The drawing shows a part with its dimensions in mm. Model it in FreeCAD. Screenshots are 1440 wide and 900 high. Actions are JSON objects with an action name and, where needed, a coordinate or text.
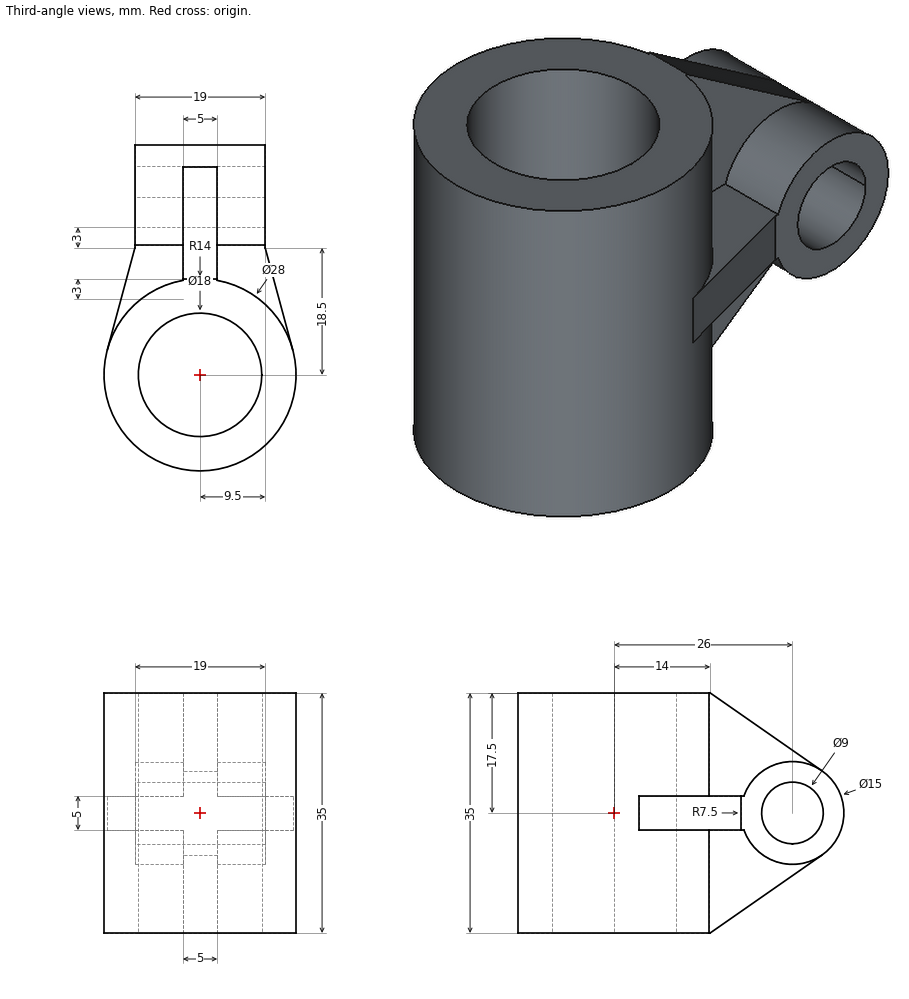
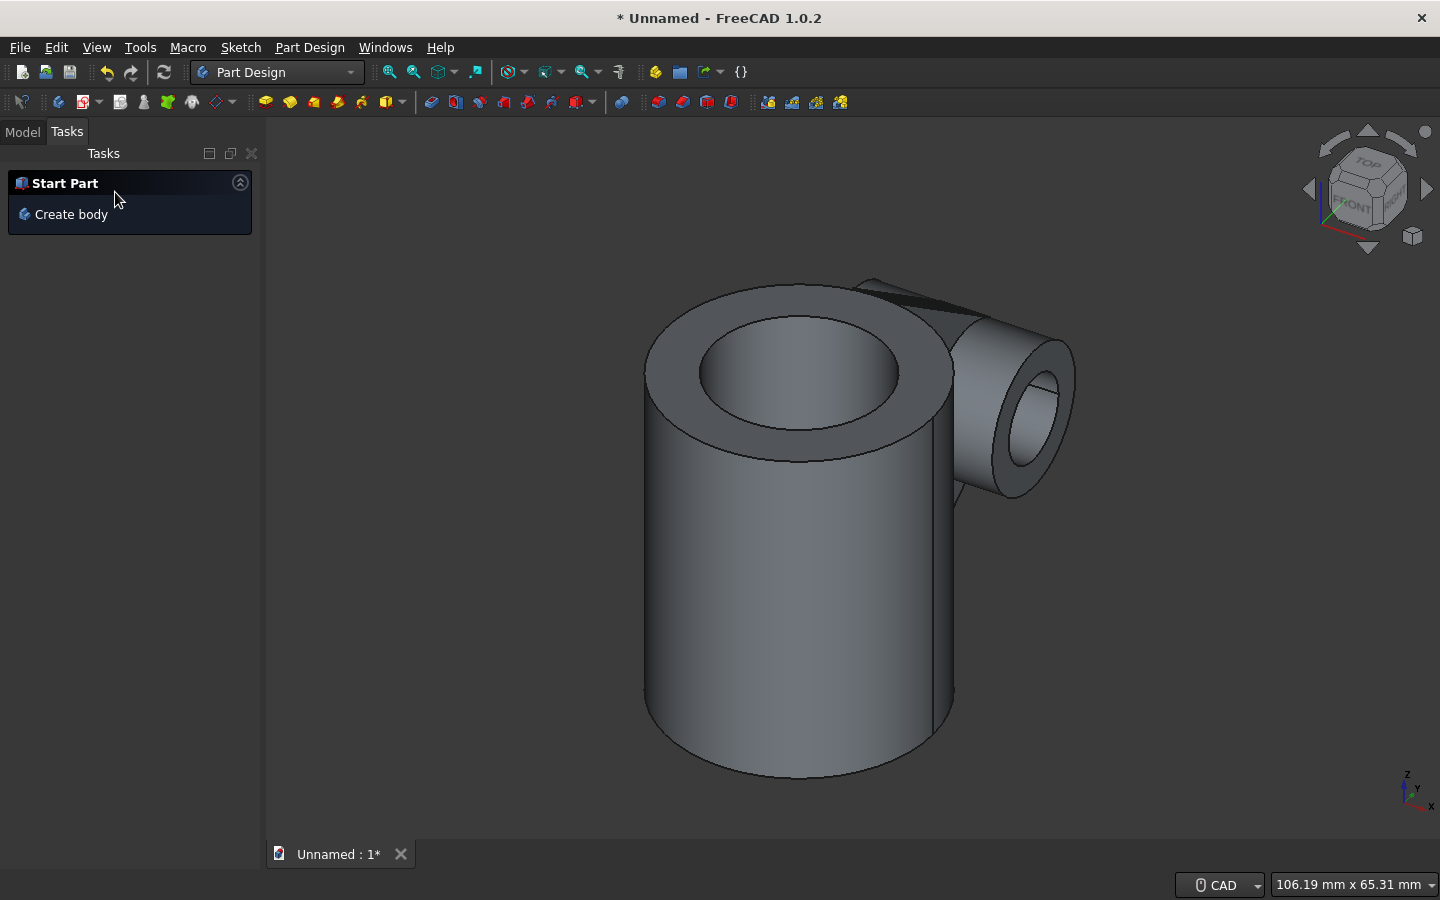
{"action": "left_click", "coordinate": [60, 102]}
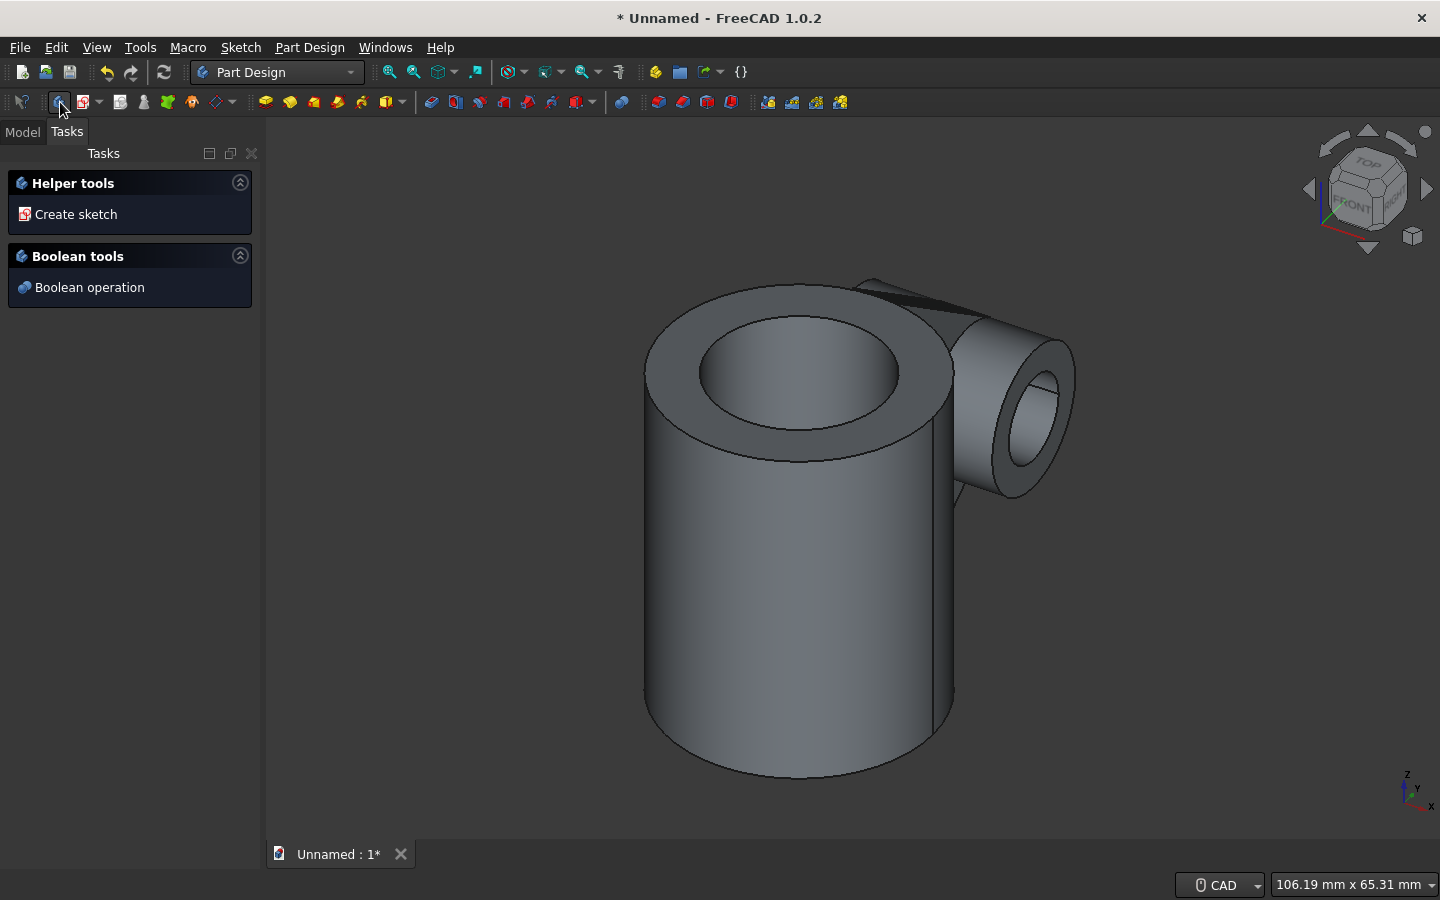
{"action": "left_click", "coordinate": [306, 799]}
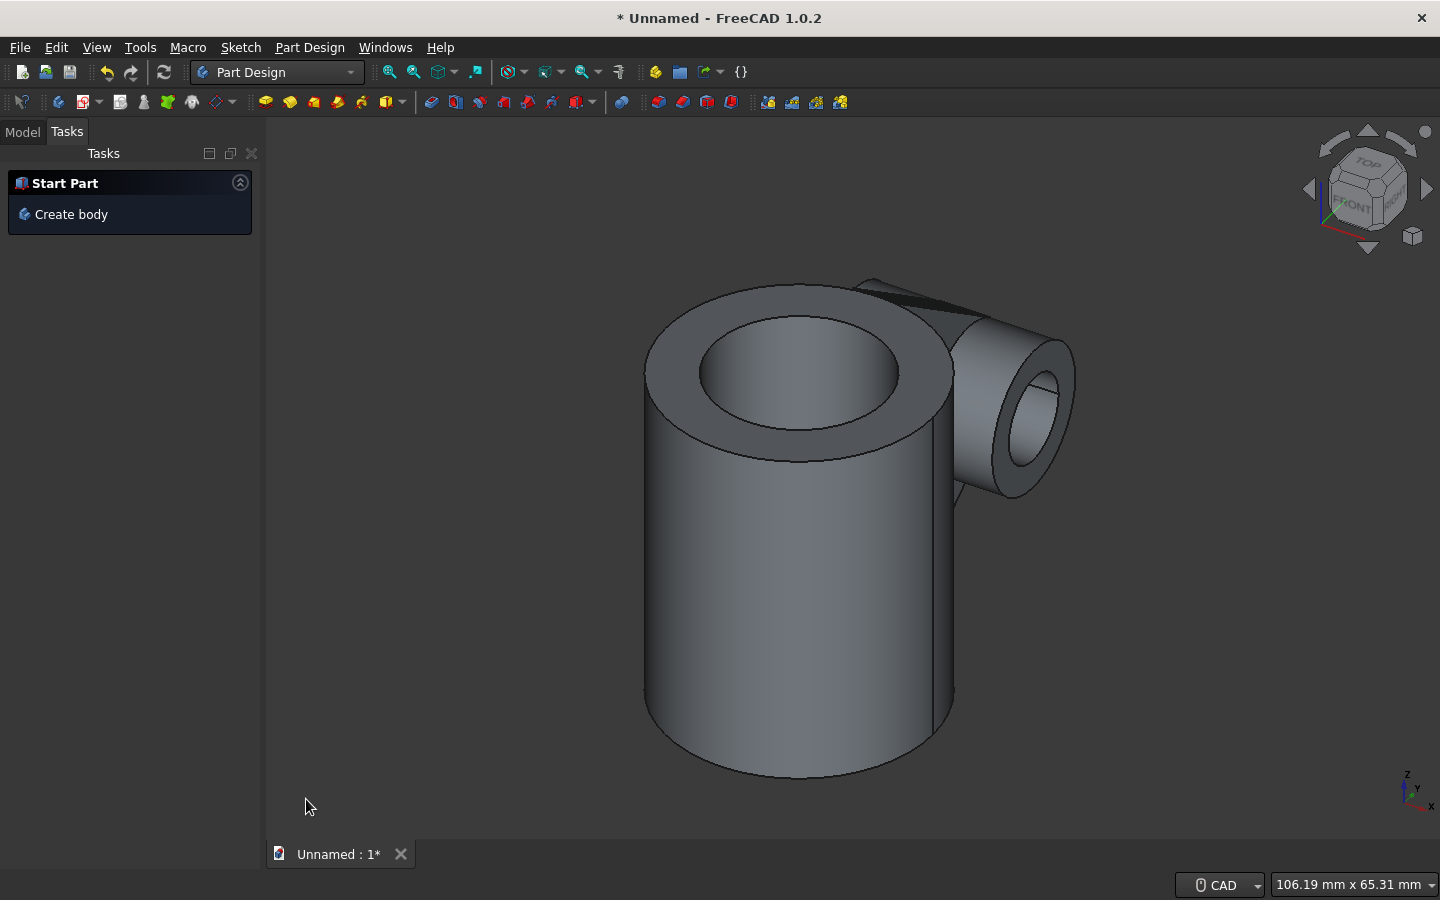
{"action": "left_click", "coordinate": [84, 102]}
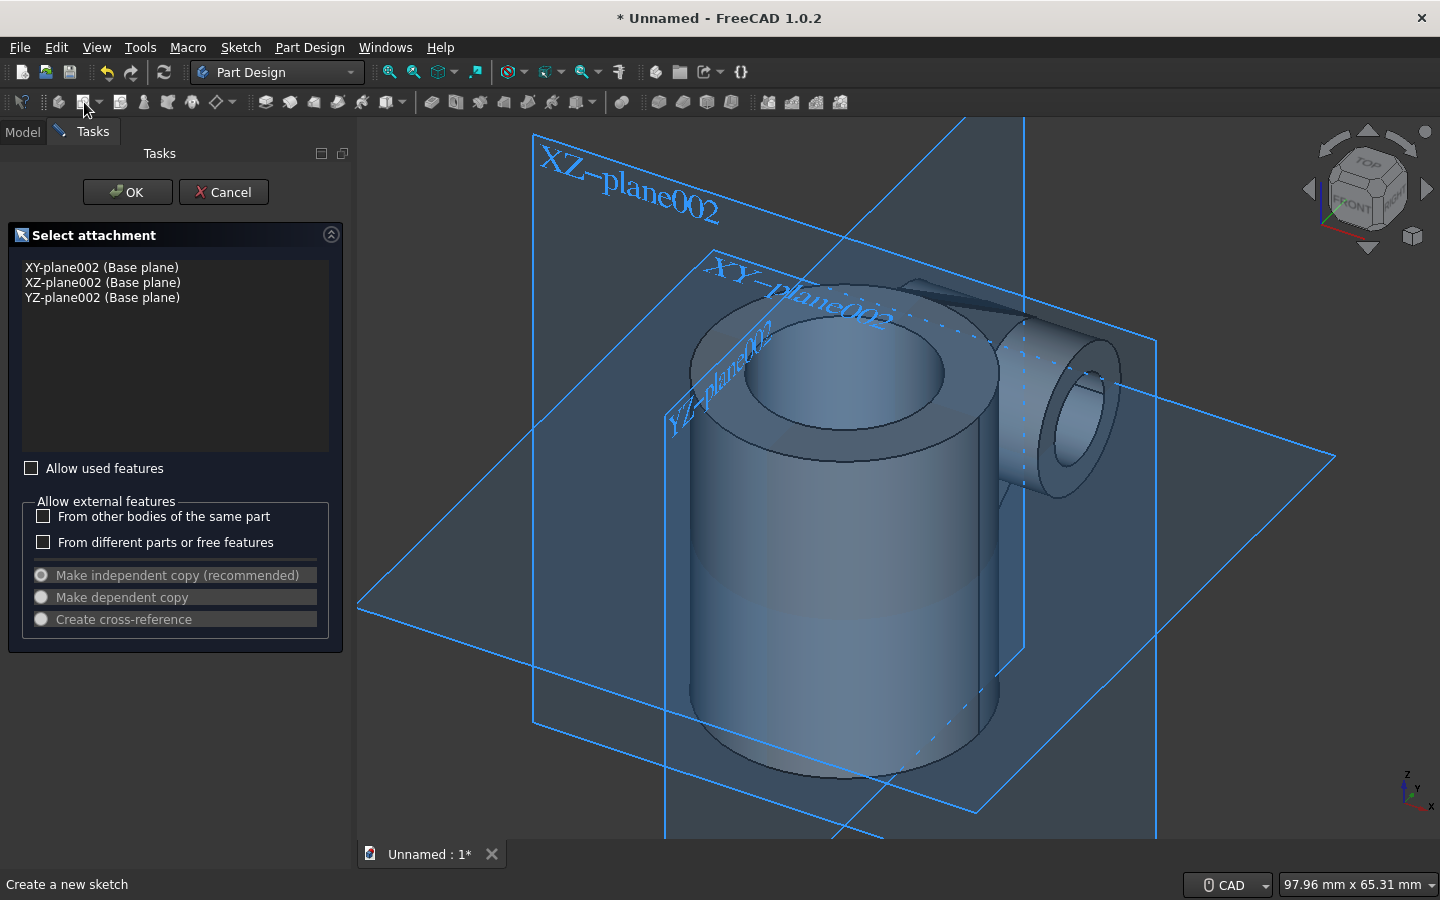
{"action": "left_click", "coordinate": [82, 268]}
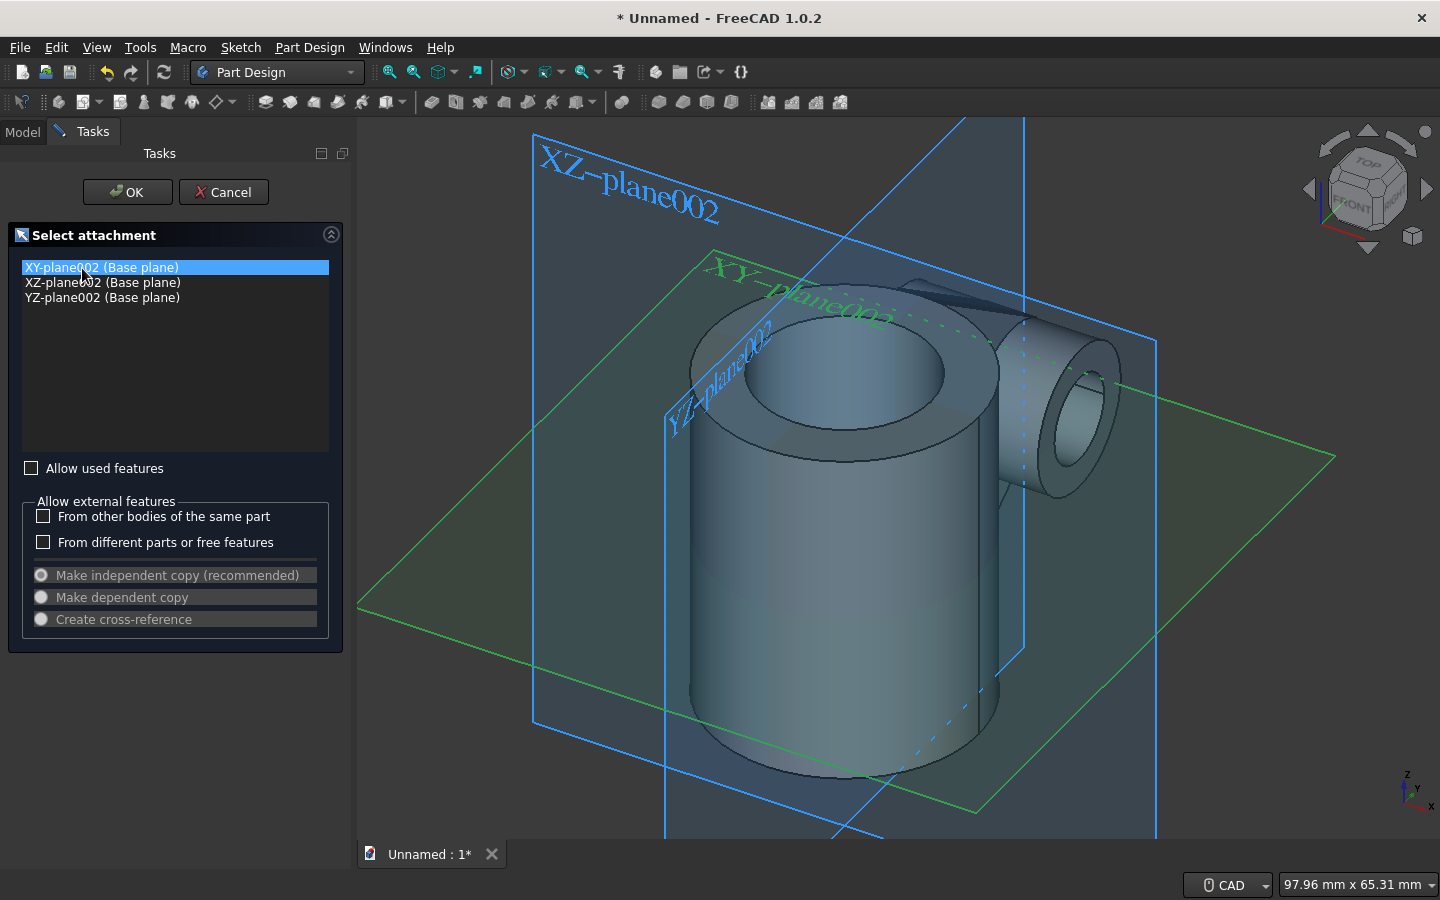
{"action": "left_click", "coordinate": [128, 192]}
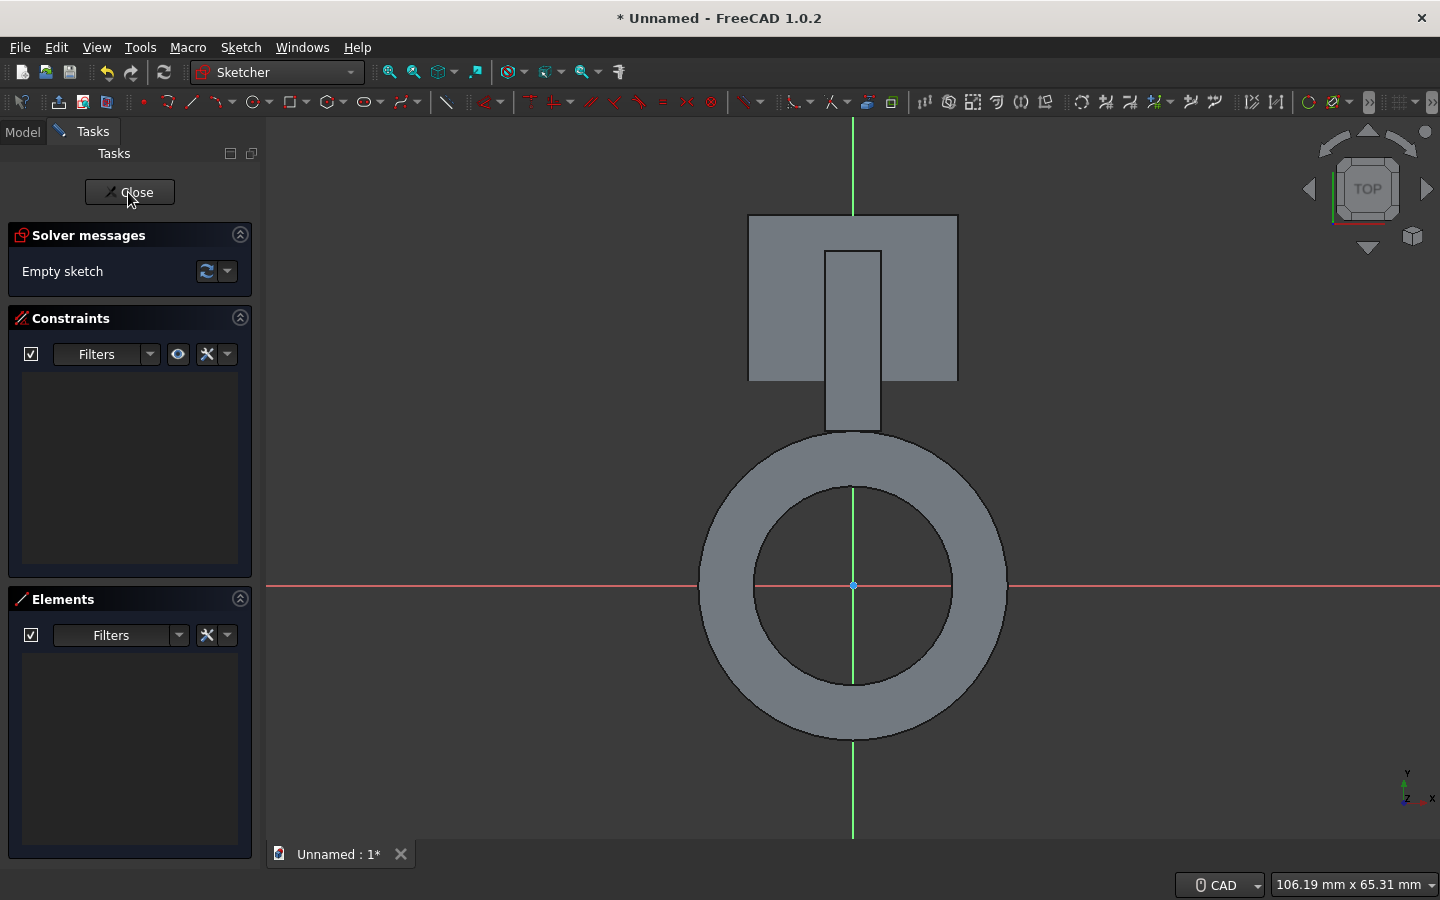
{"action": "scroll", "coordinate": [909, 488], "scroll_direction": "up", "scroll_amount": 4}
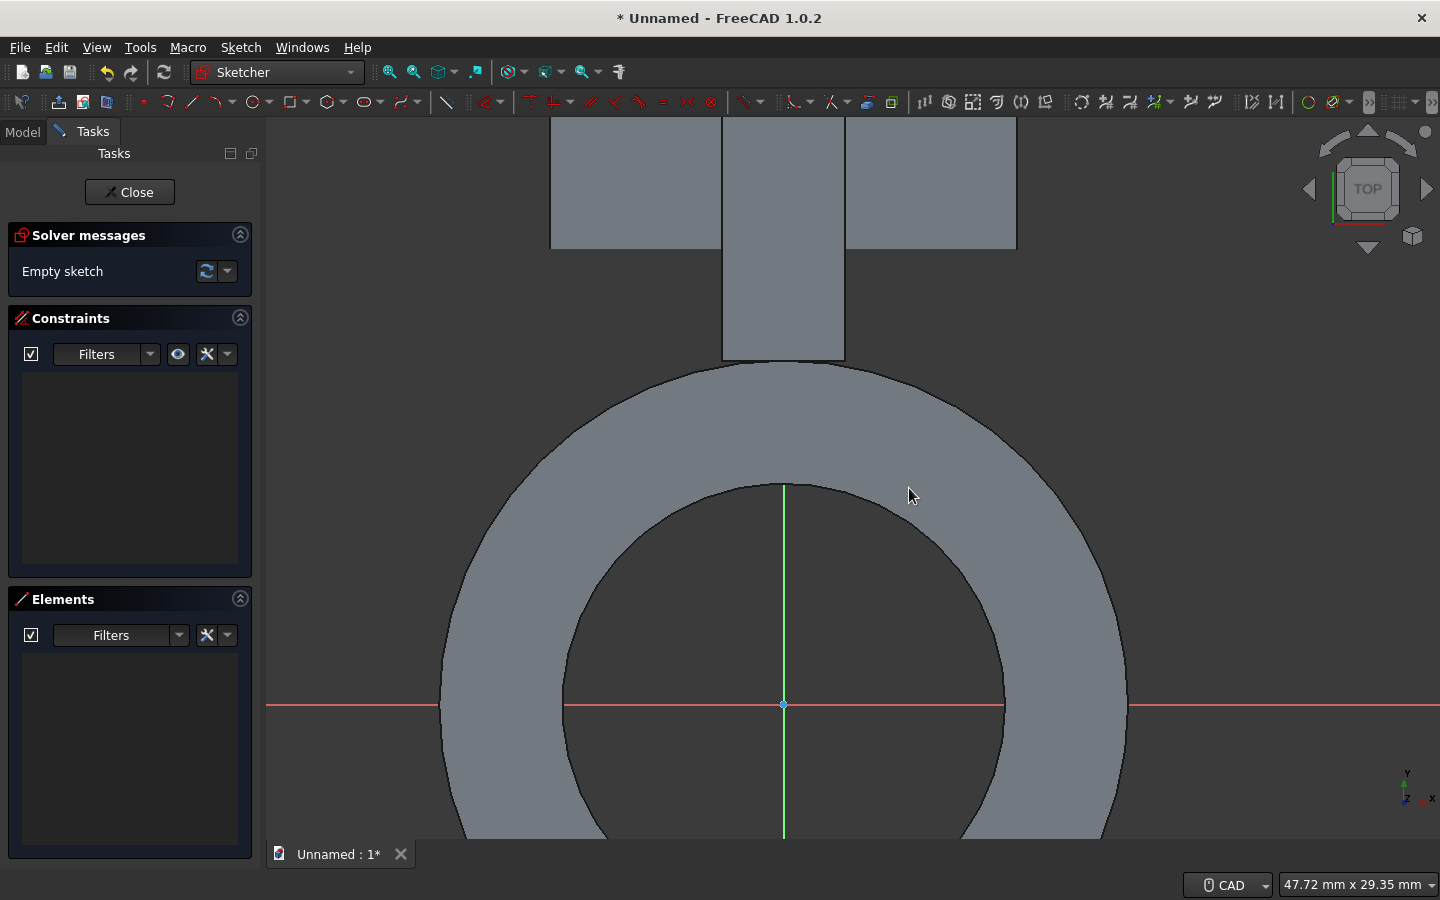
{"action": "left_click", "coordinate": [168, 102]}